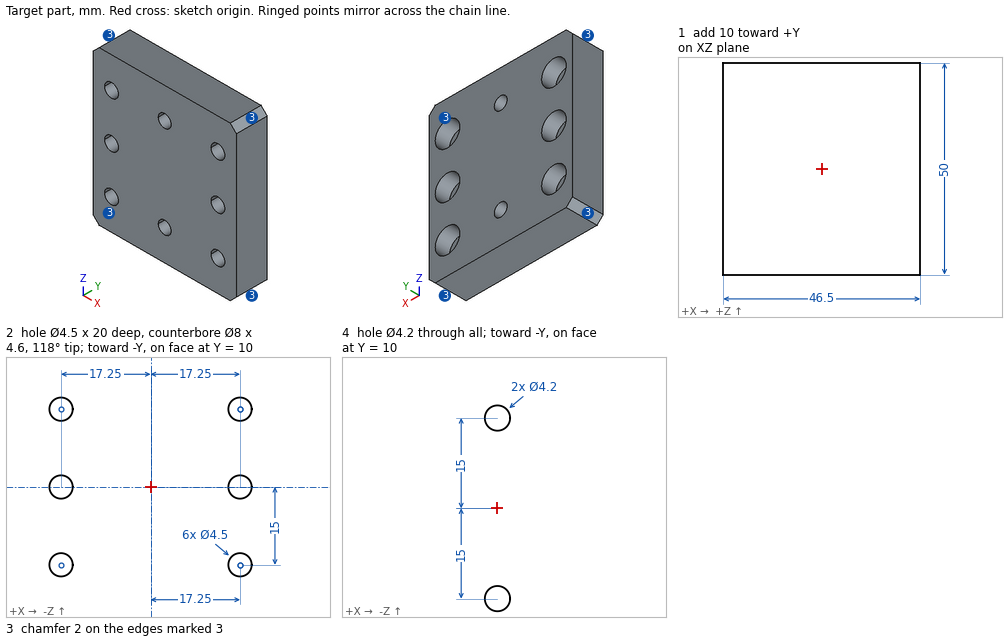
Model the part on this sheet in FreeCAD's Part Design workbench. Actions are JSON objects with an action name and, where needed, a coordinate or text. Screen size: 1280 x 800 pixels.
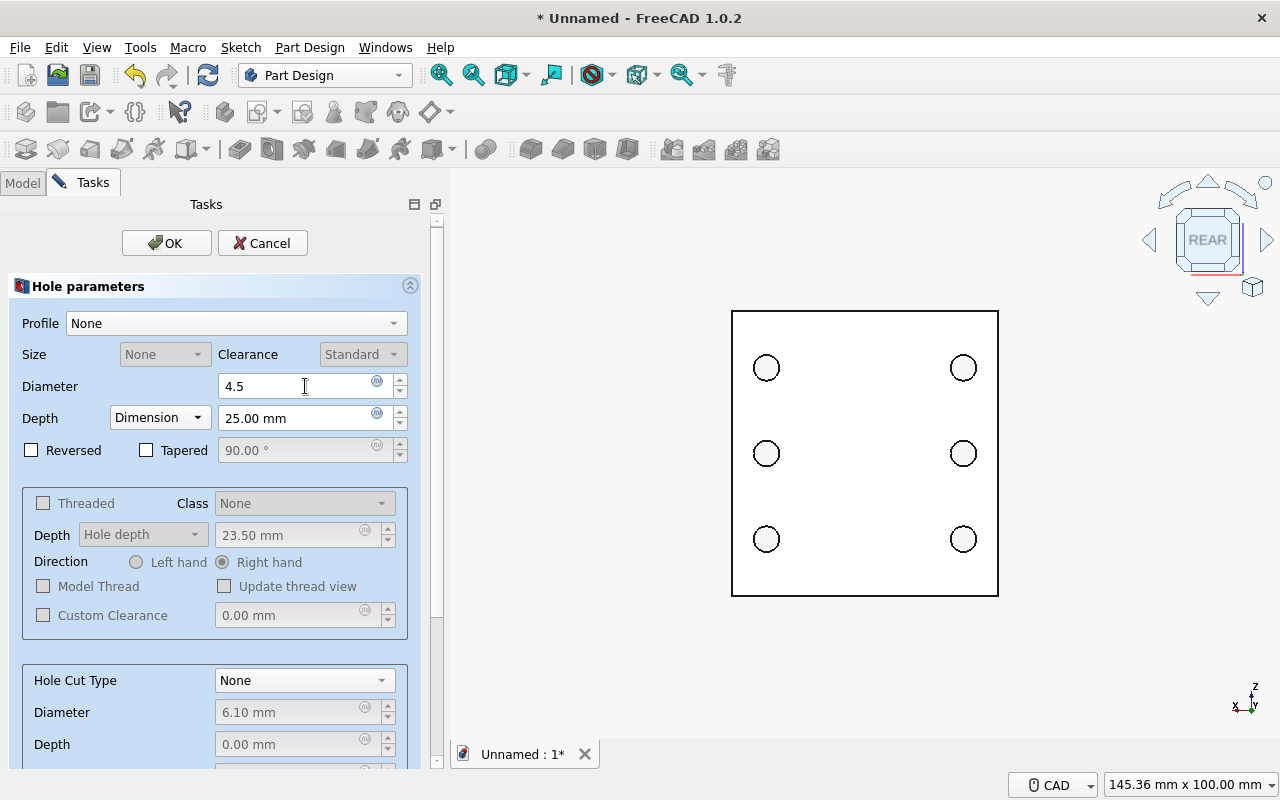
{"action": "triple_click", "coordinate": [305, 418]}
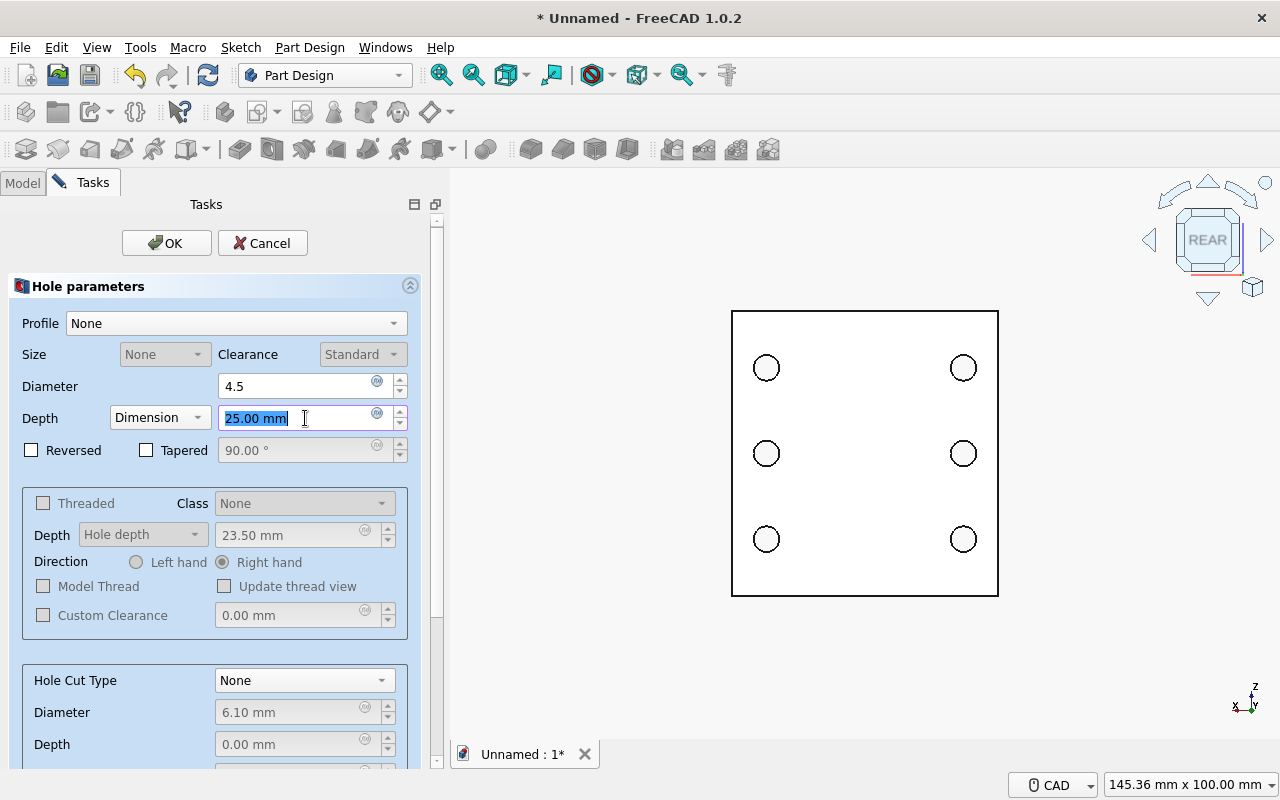
{"action": "type", "text": "20"}
{"action": "key", "text": "Tab"}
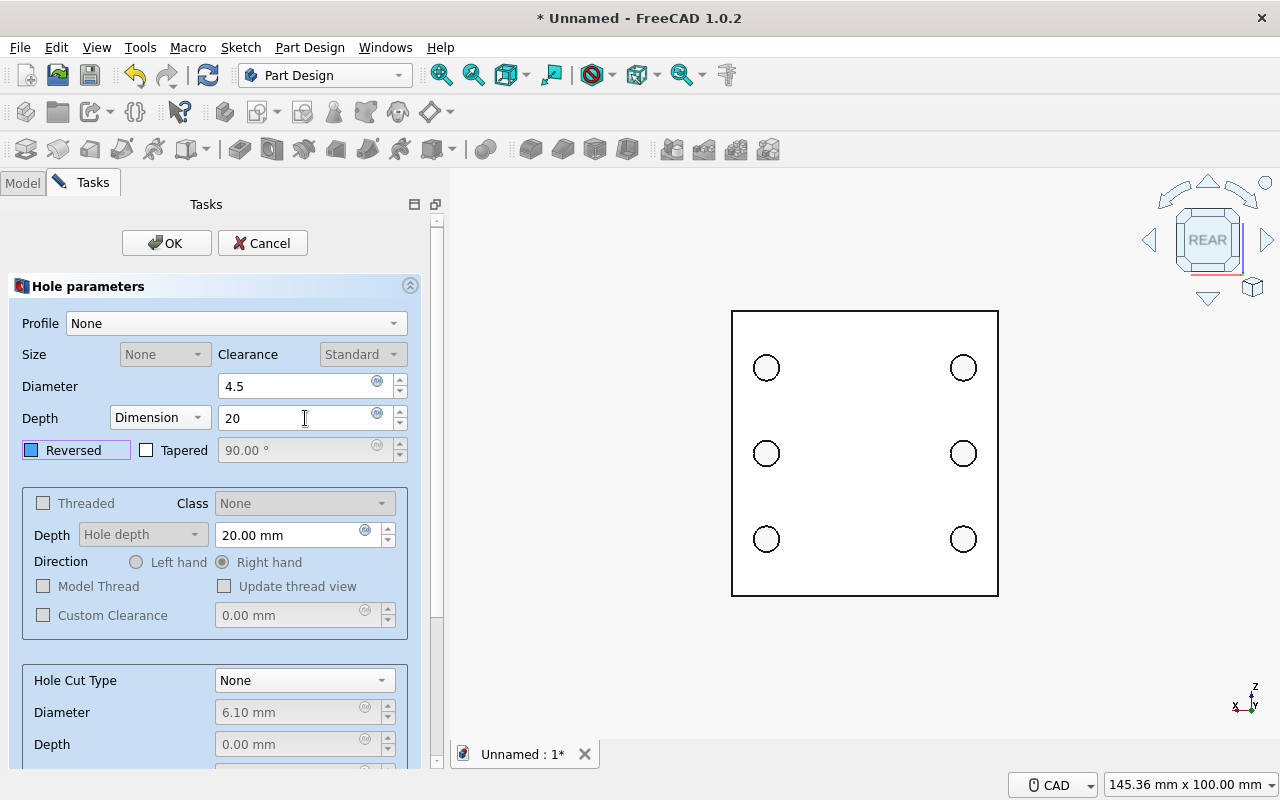
{"action": "left_click", "coordinate": [306, 680]}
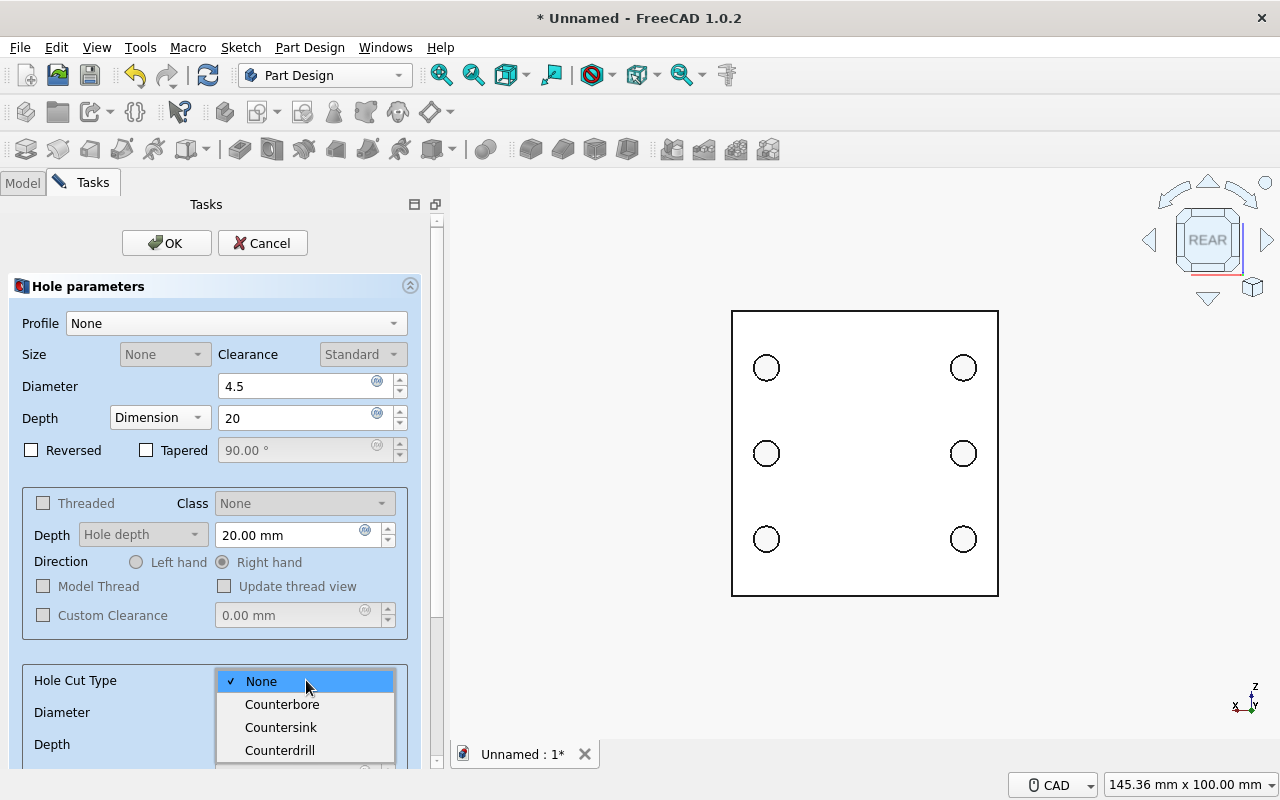
{"action": "left_click", "coordinate": [304, 704]}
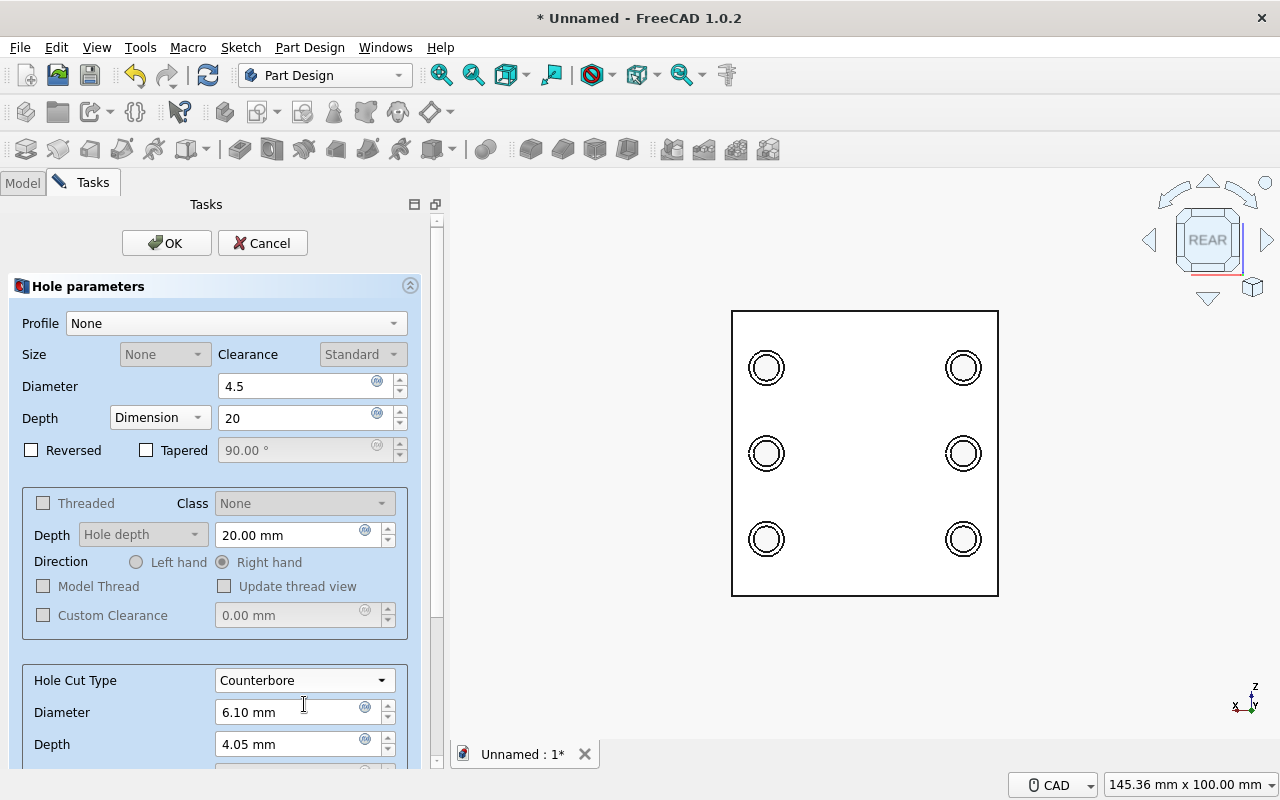
{"action": "triple_click", "coordinate": [298, 712]}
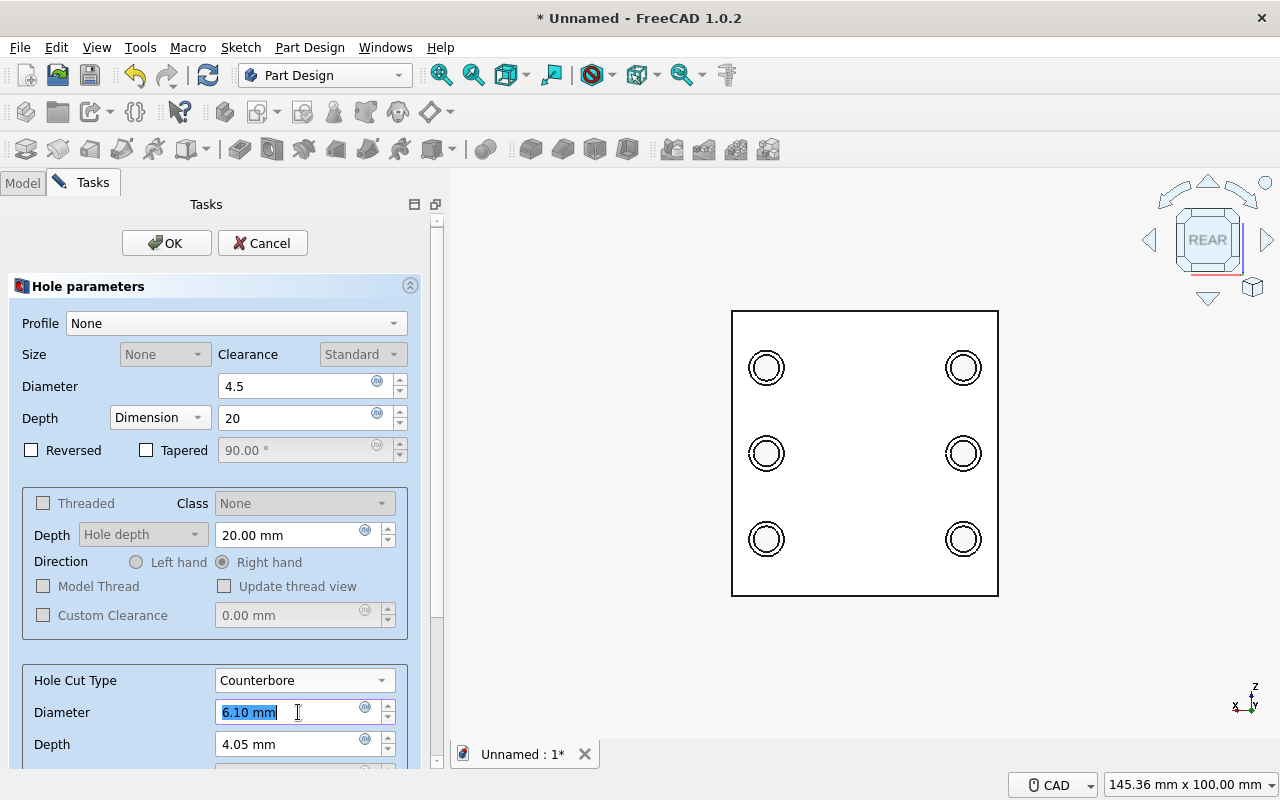
{"action": "type", "text": "8"}
{"action": "key", "text": "Tab"}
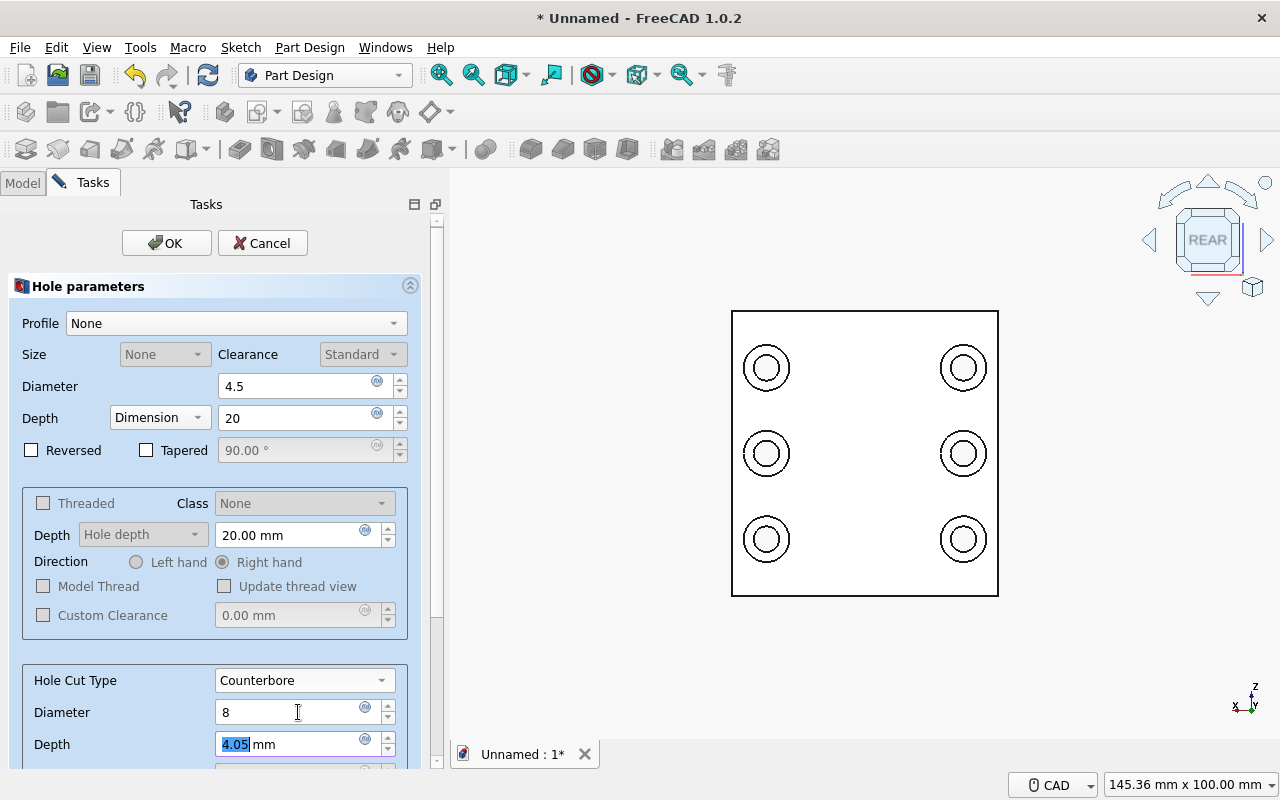
{"action": "type", "text": "4.6"}
{"action": "key", "text": "Tab"}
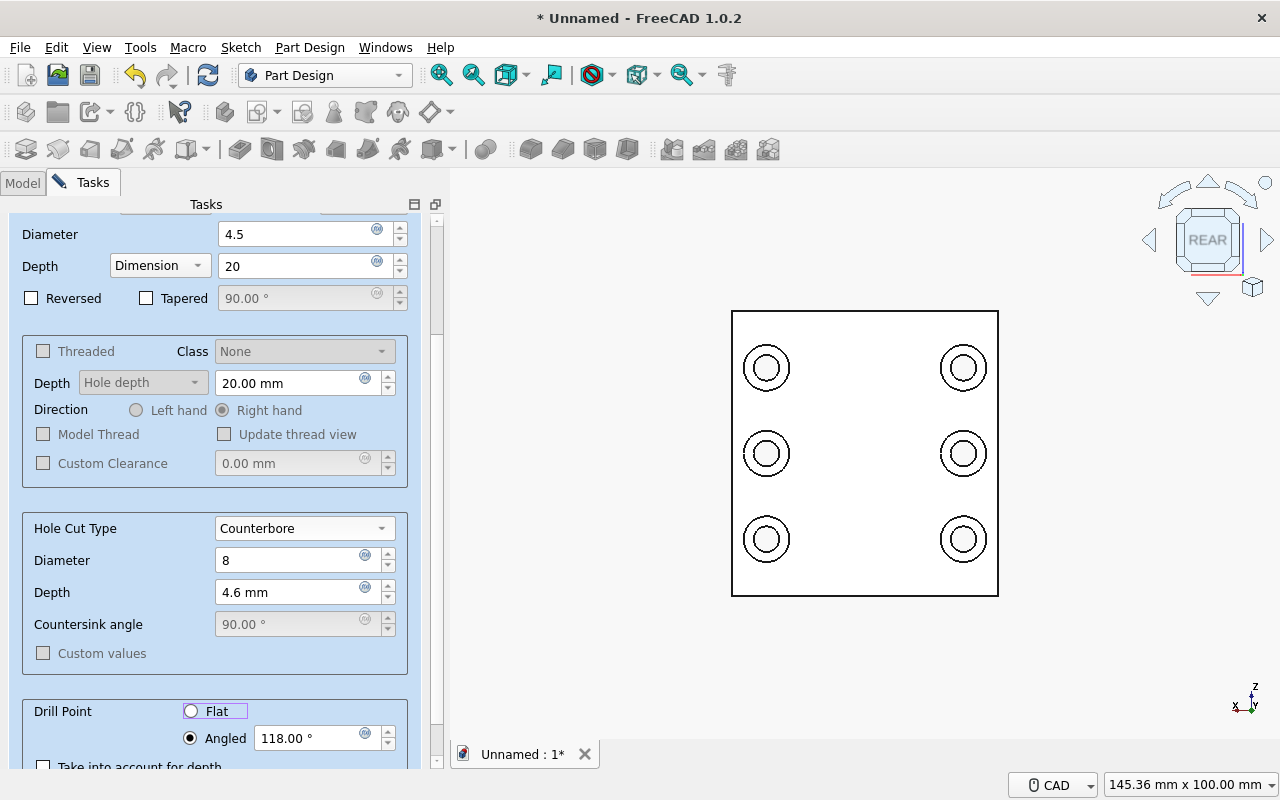
{"action": "scroll", "coordinate": [437, 491], "scroll_direction": "up", "scroll_amount": 4}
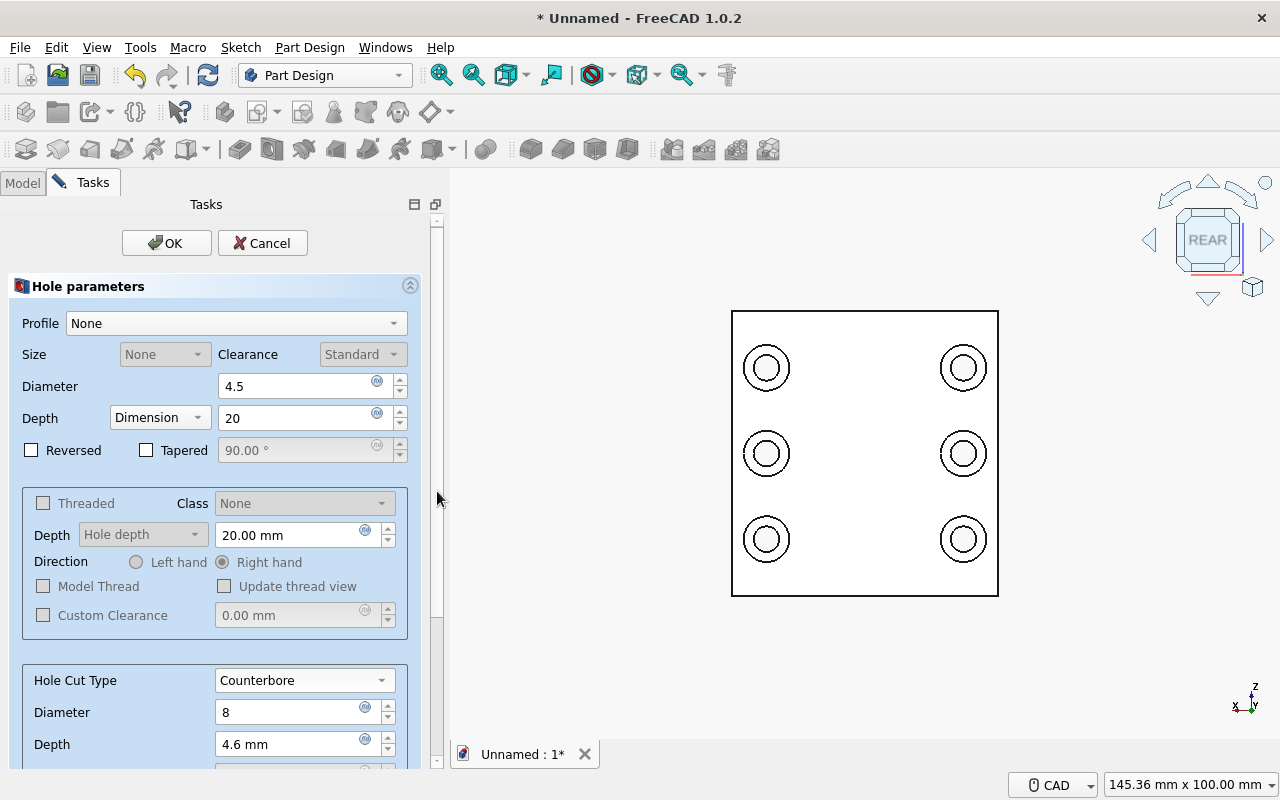
{"action": "left_click", "coordinate": [167, 243]}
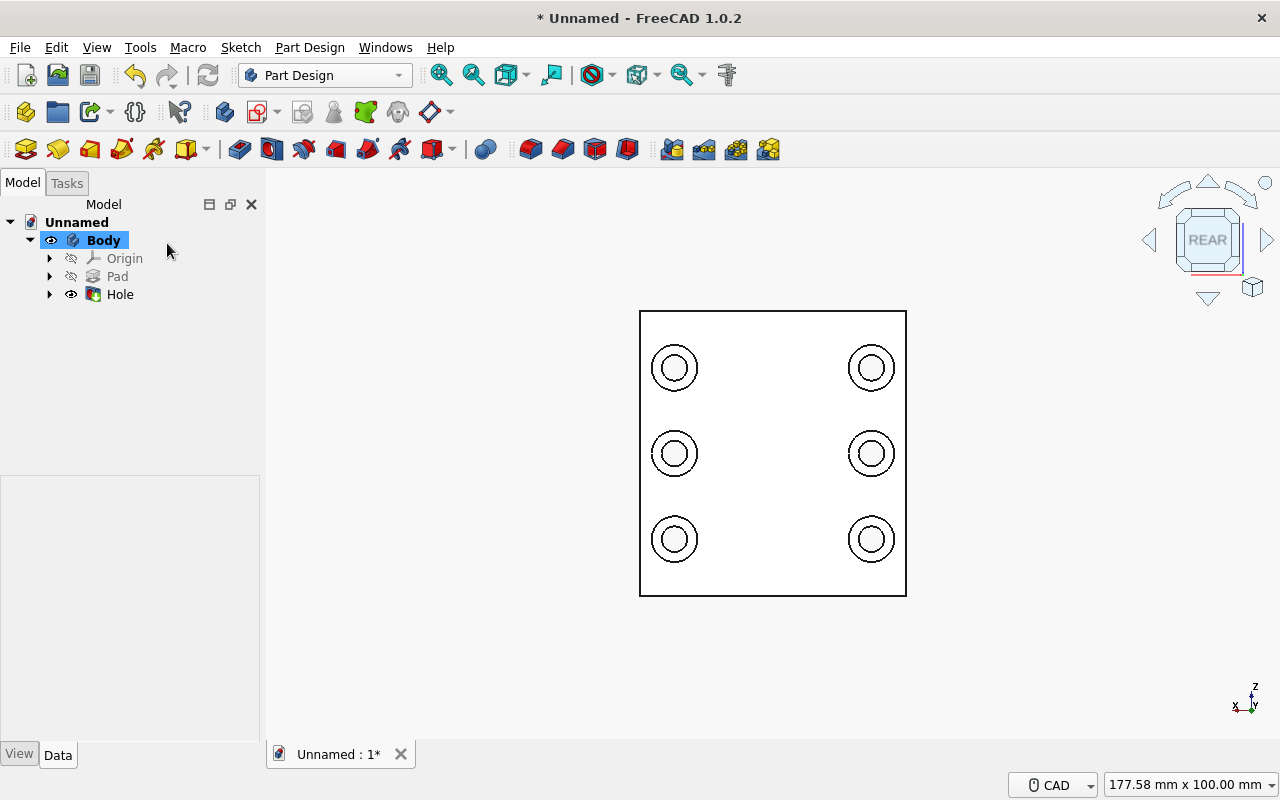
{"action": "key", "text": "0"}